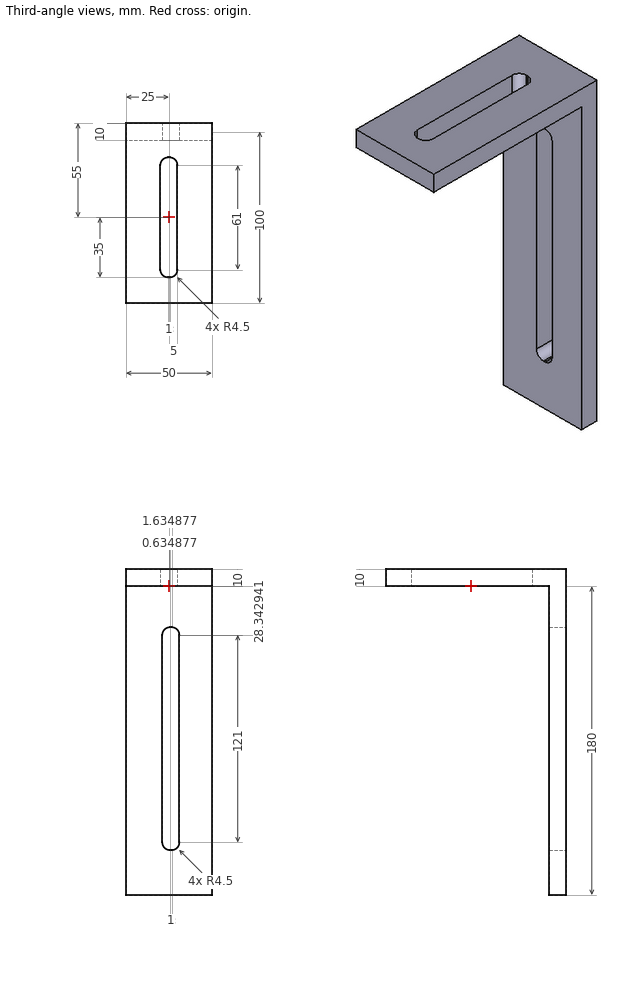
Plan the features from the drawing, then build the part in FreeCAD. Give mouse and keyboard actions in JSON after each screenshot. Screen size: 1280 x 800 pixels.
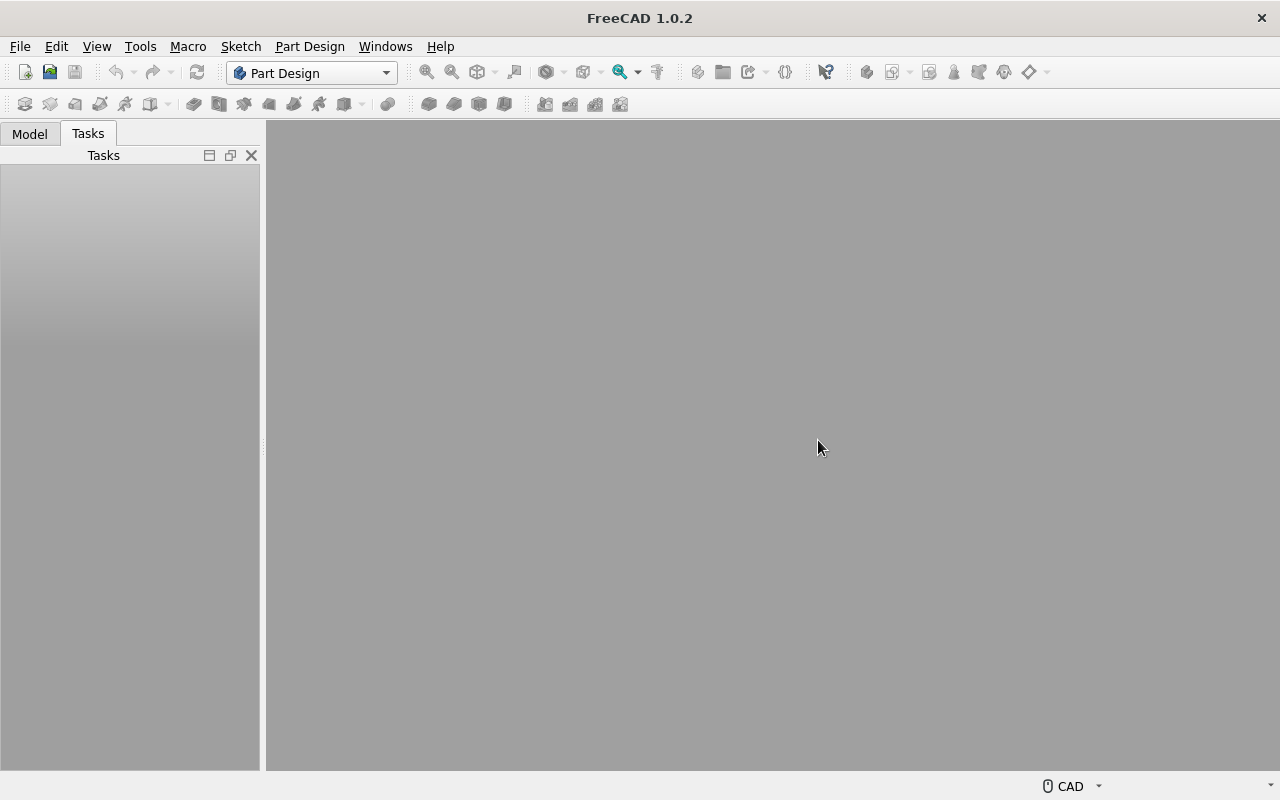
{"action": "left_click", "coordinate": [25, 72]}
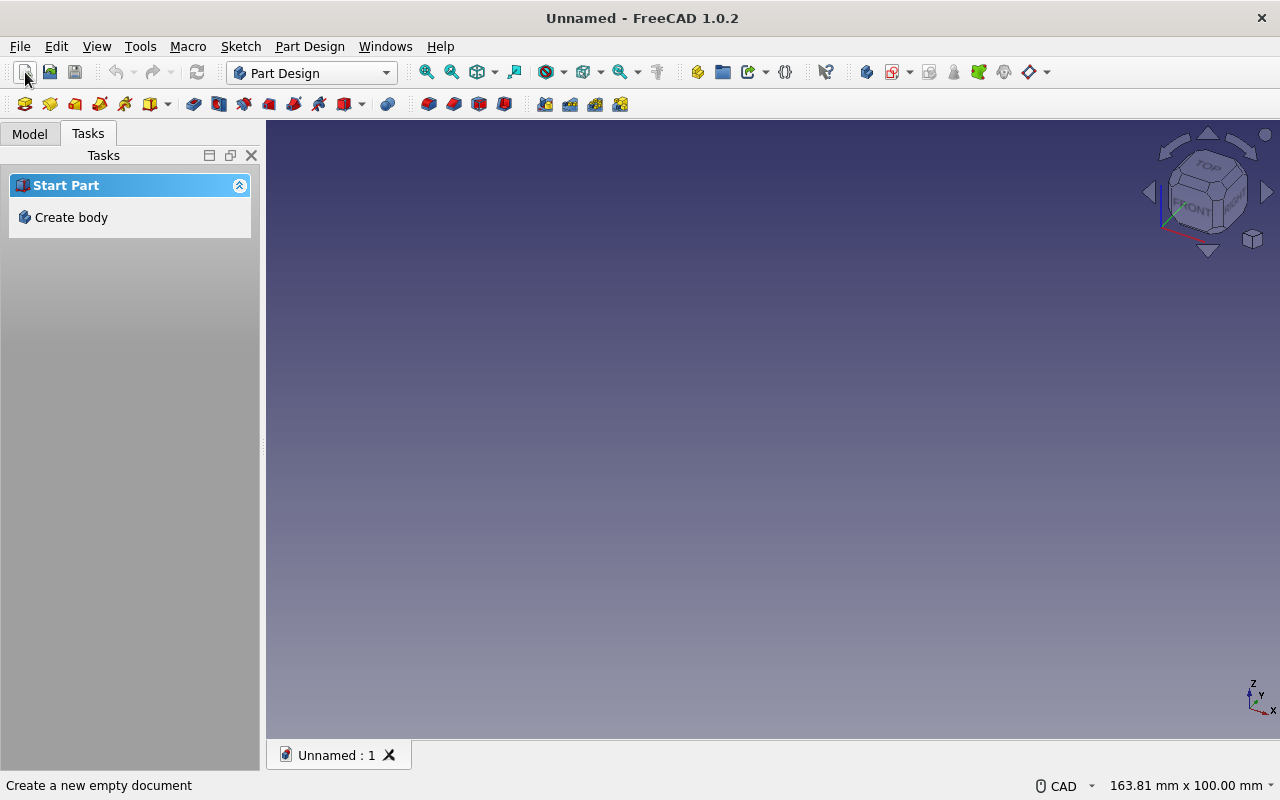
{"action": "left_click", "coordinate": [892, 72]}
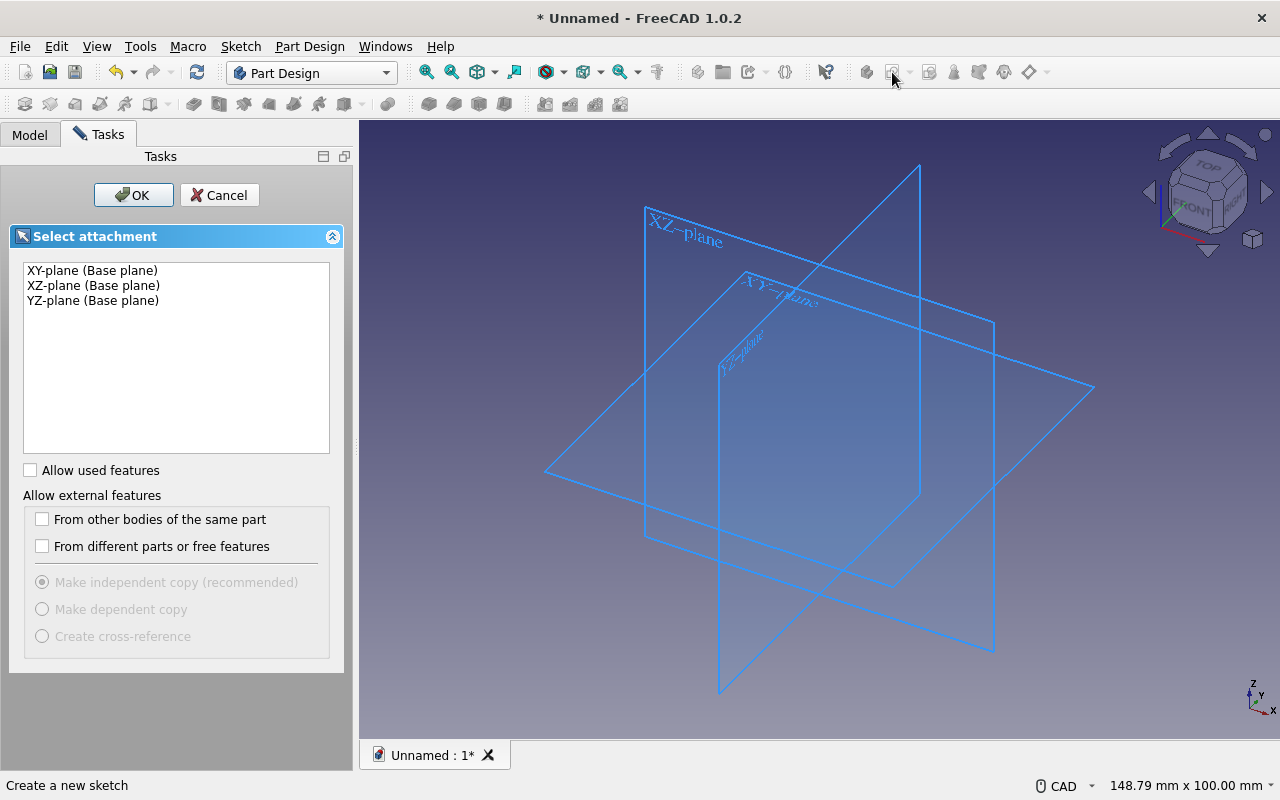
{"action": "left_click", "coordinate": [84, 270]}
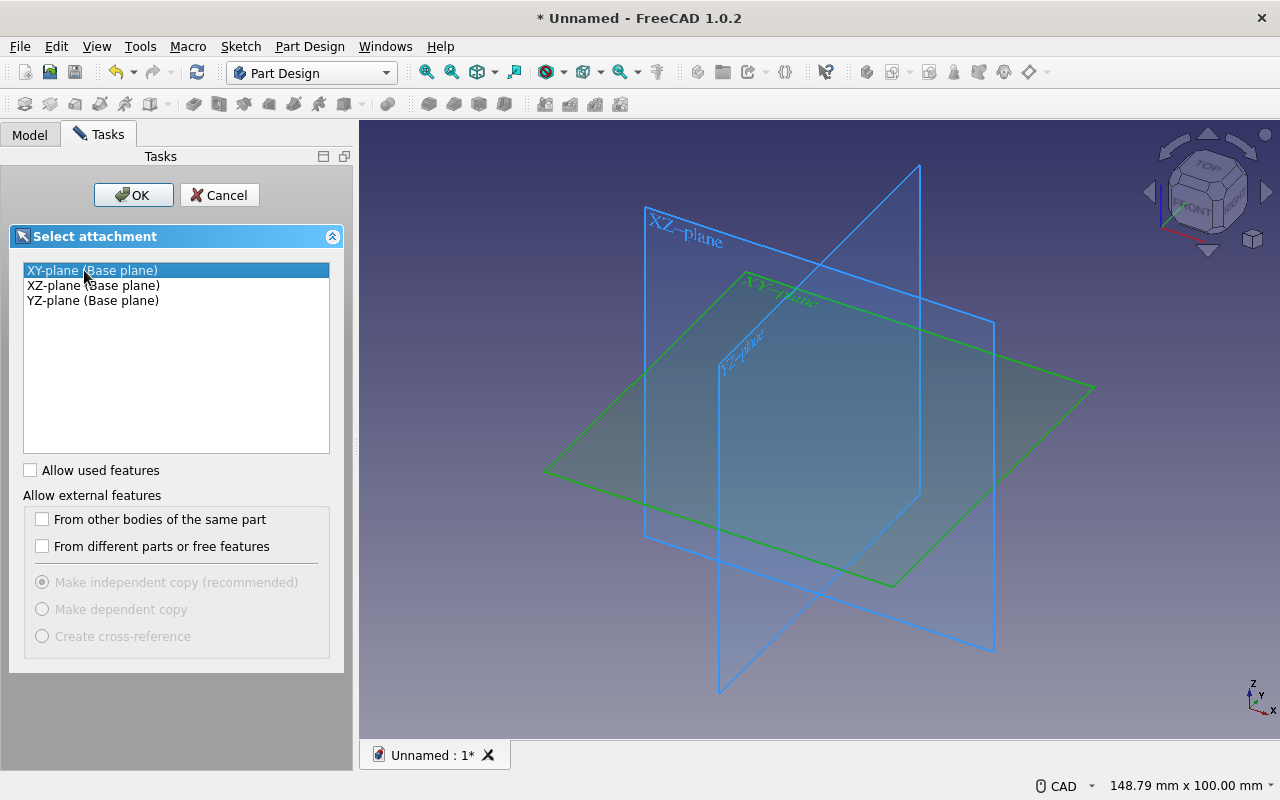
{"action": "left_click", "coordinate": [134, 195]}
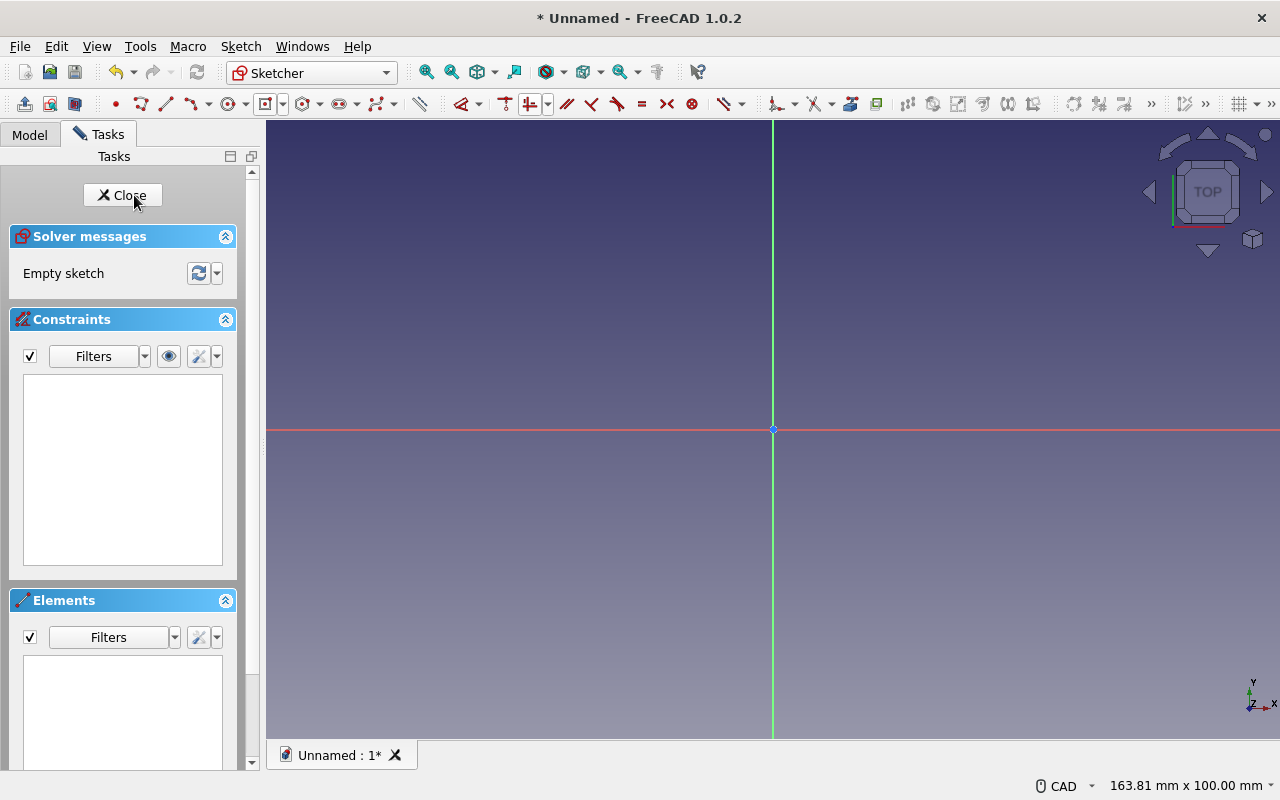
{"action": "scroll", "coordinate": [565, 429], "scroll_direction": "down", "scroll_amount": 2}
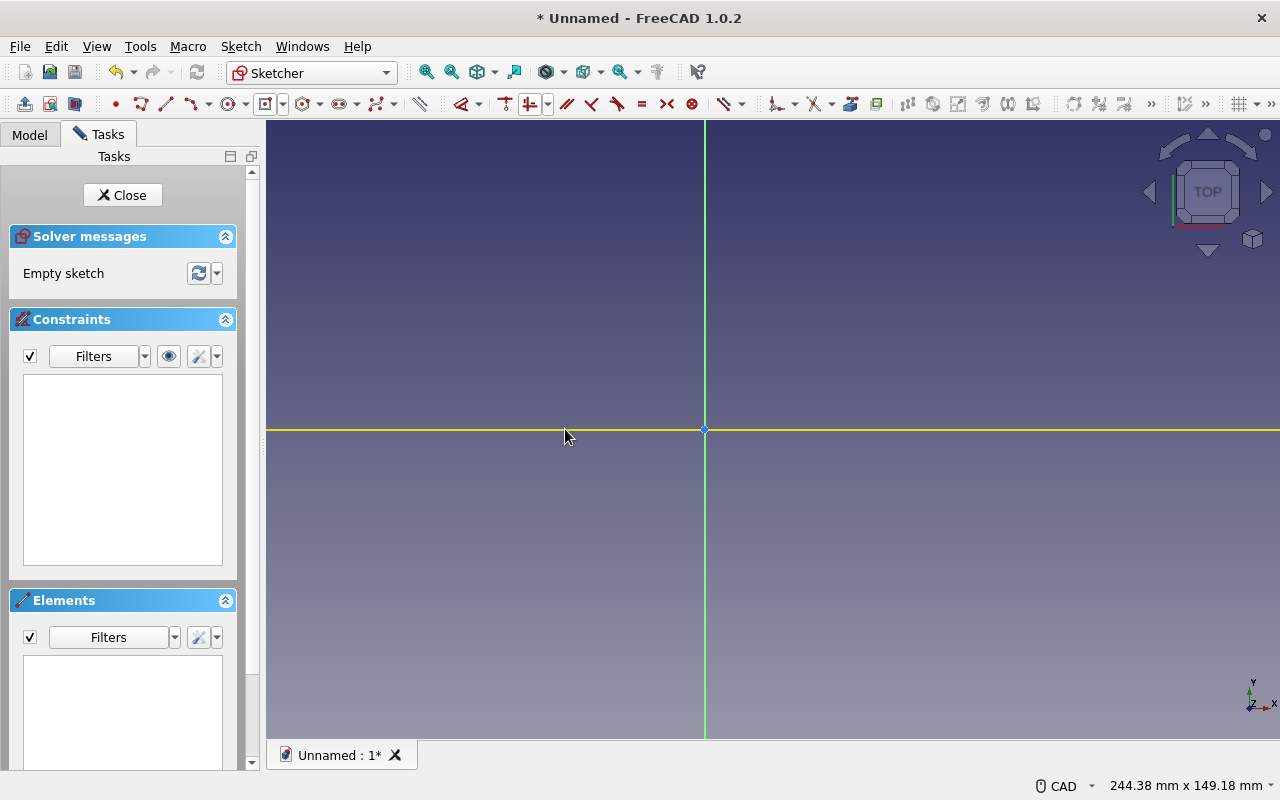
{"action": "left_click", "coordinate": [264, 104]}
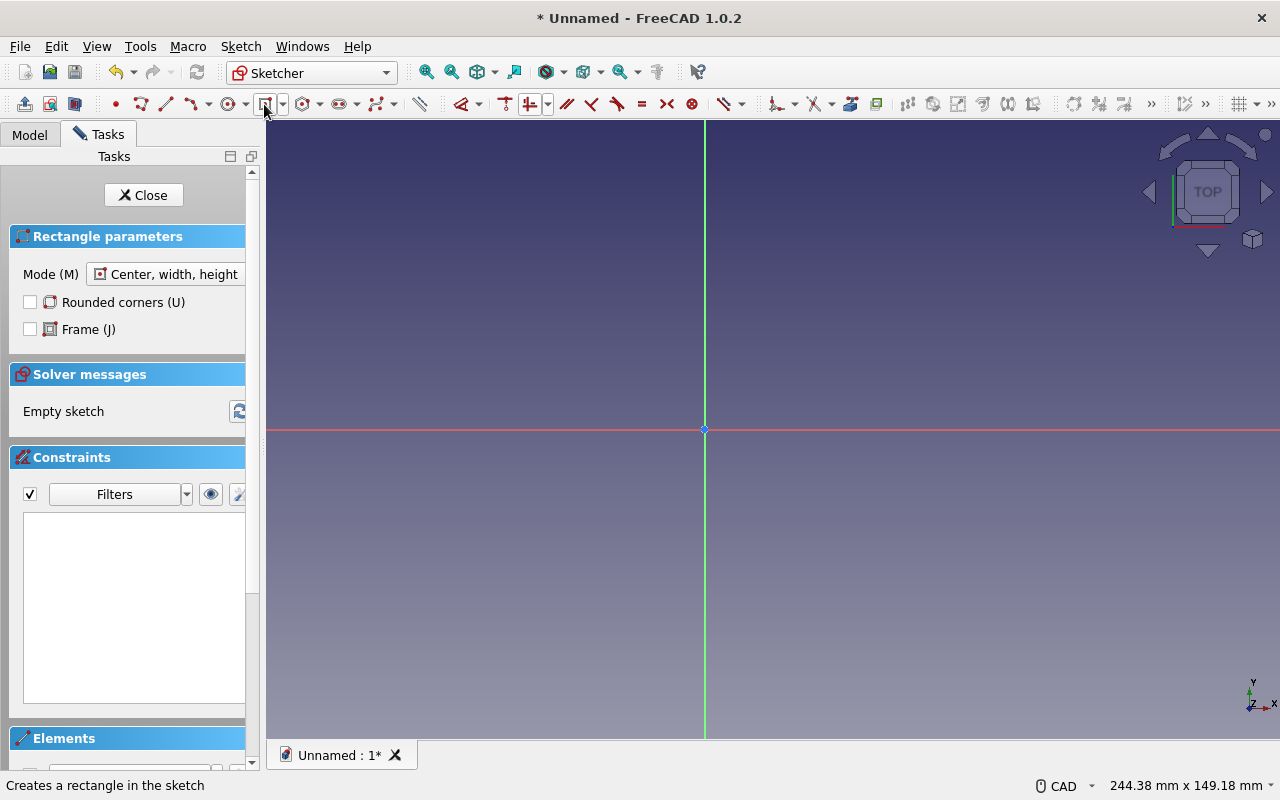
{"action": "left_click", "coordinate": [705, 430]}
{"action": "left_click", "coordinate": [808, 222]}
{"action": "key", "text": "Escape"}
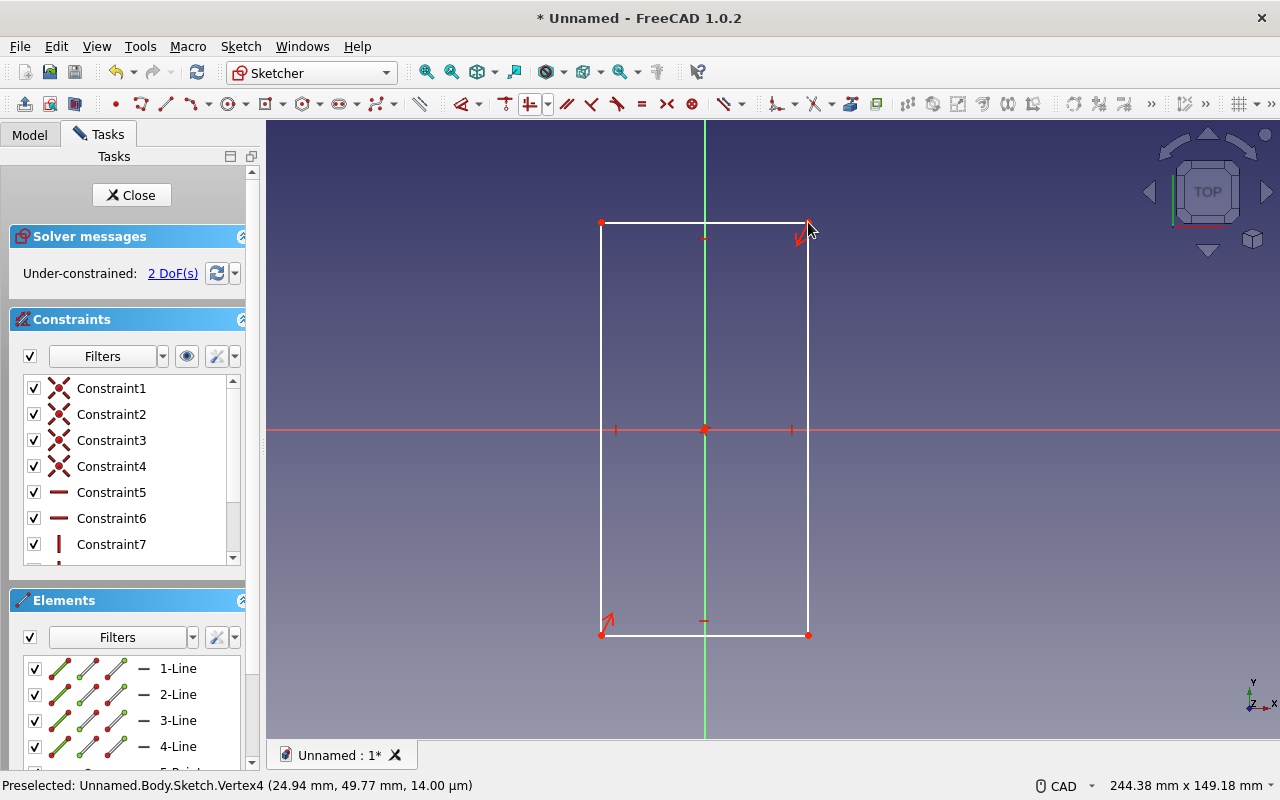
{"action": "left_click", "coordinate": [460, 104]}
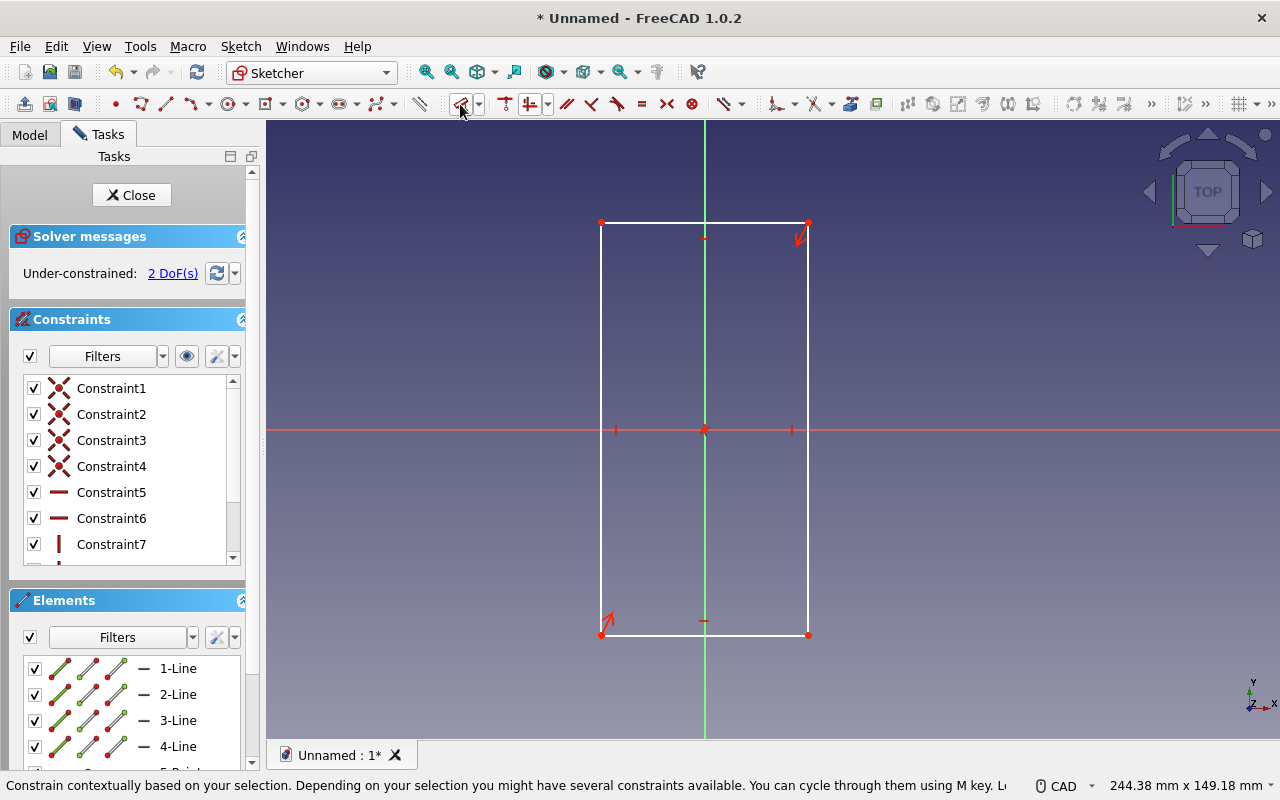
{"action": "left_click", "coordinate": [663, 636]}
{"action": "left_click", "coordinate": [657, 670]}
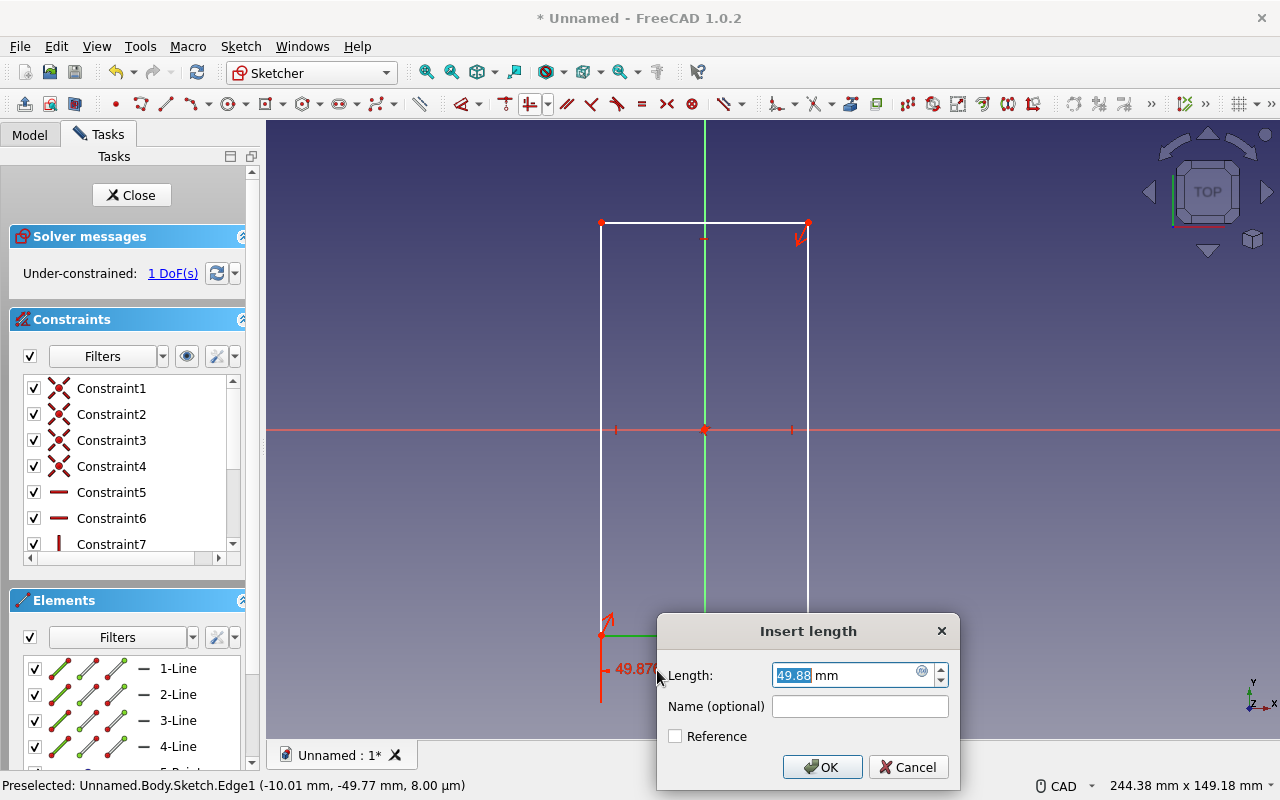
{"action": "type", "text": "50"}
{"action": "key", "text": "Return"}